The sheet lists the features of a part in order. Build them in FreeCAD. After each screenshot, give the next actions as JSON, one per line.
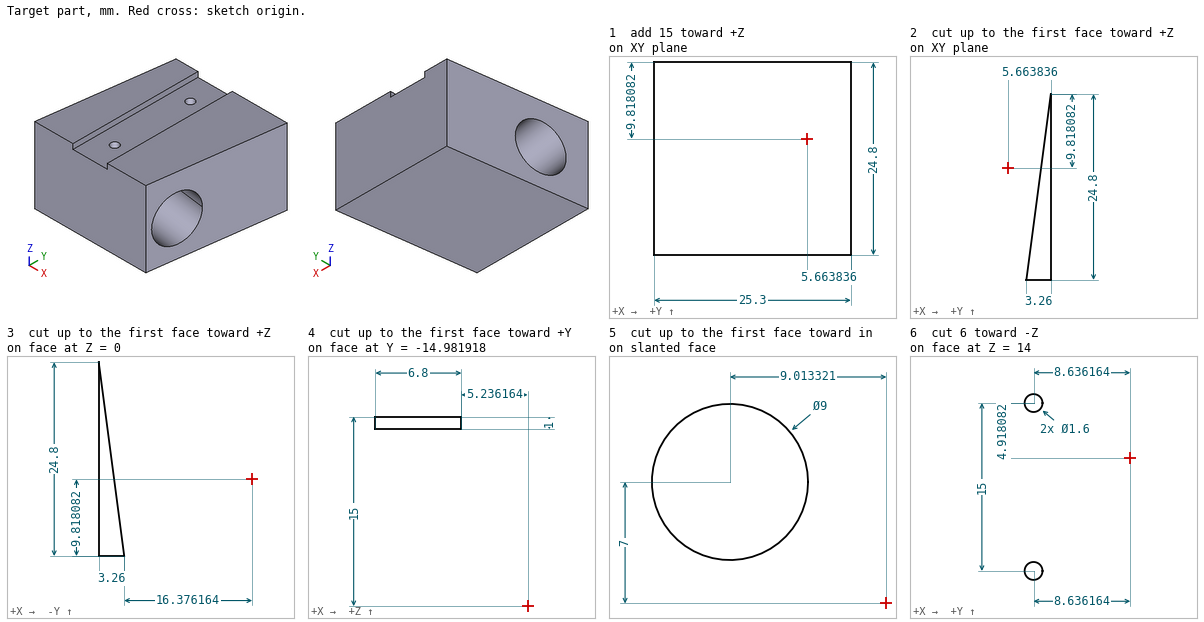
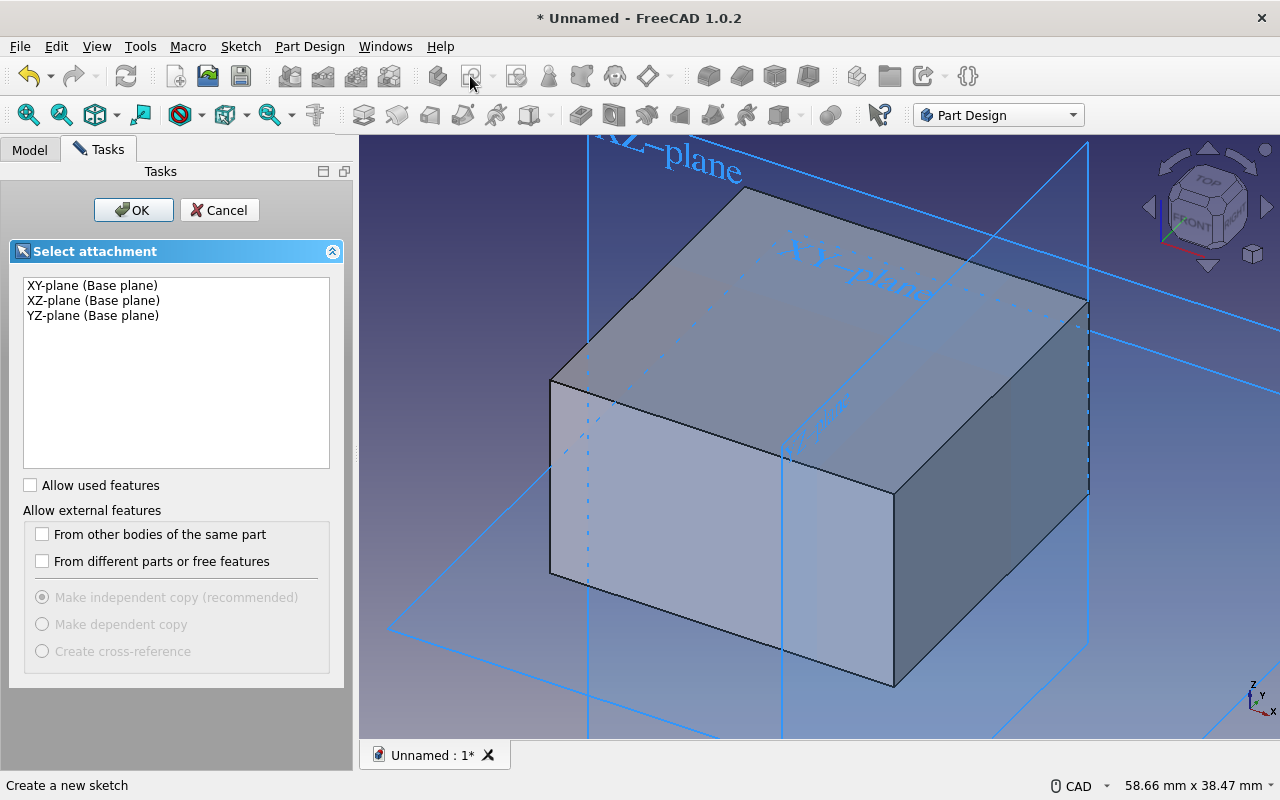
{"action": "left_click", "coordinate": [84, 286]}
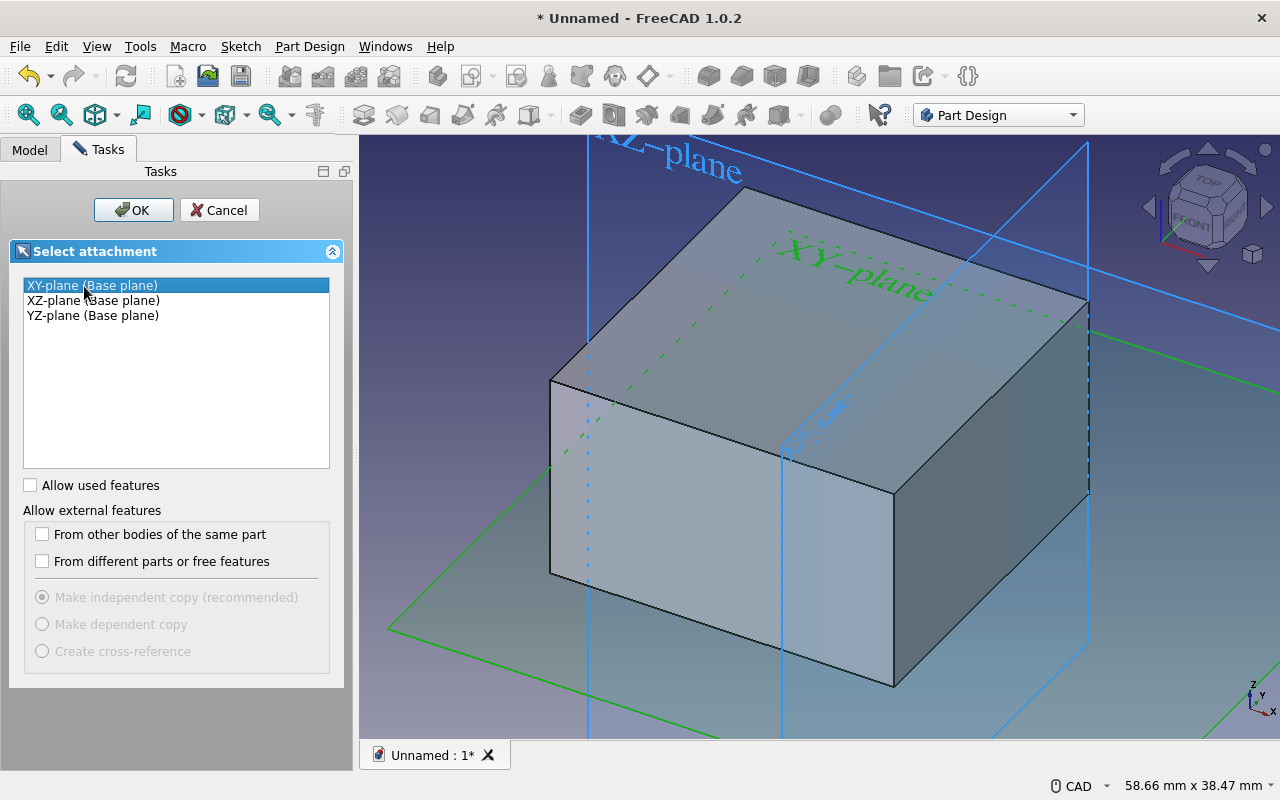
{"action": "left_click", "coordinate": [134, 210]}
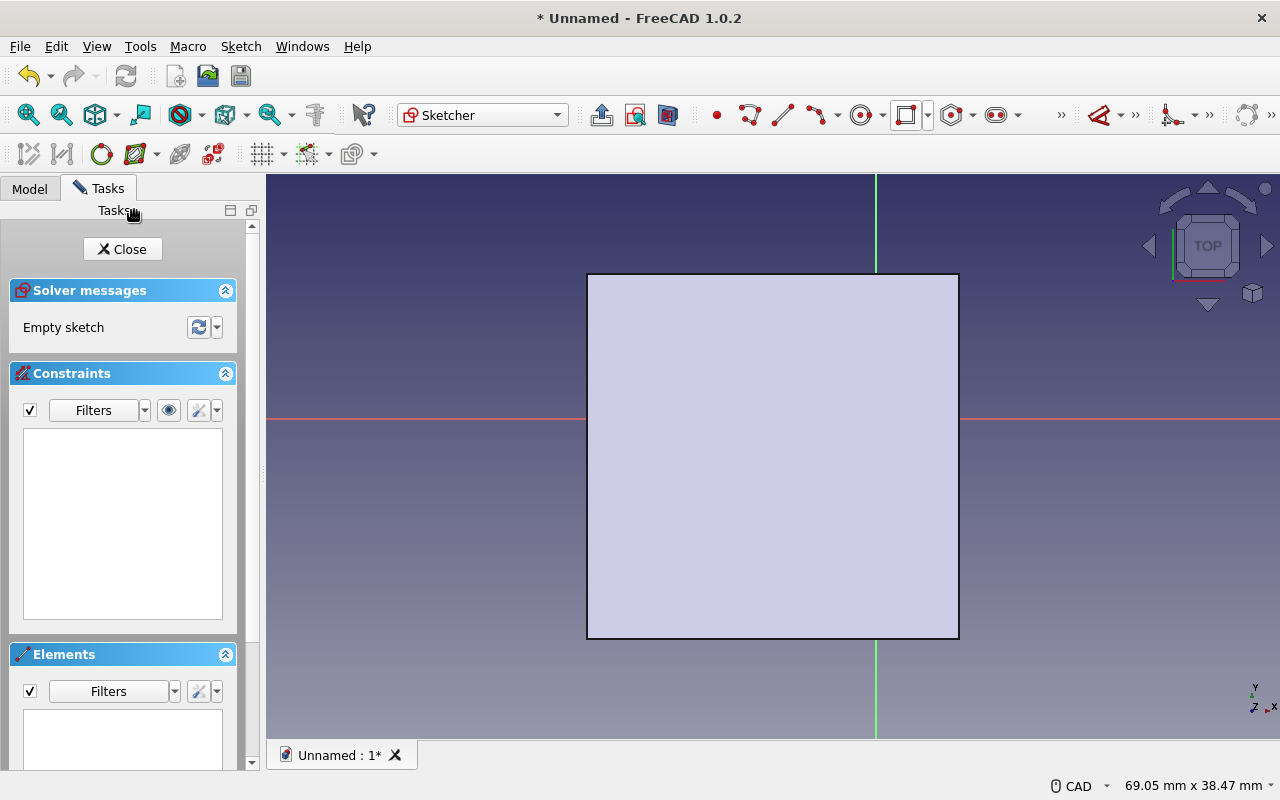
{"action": "left_click", "coordinate": [668, 116]}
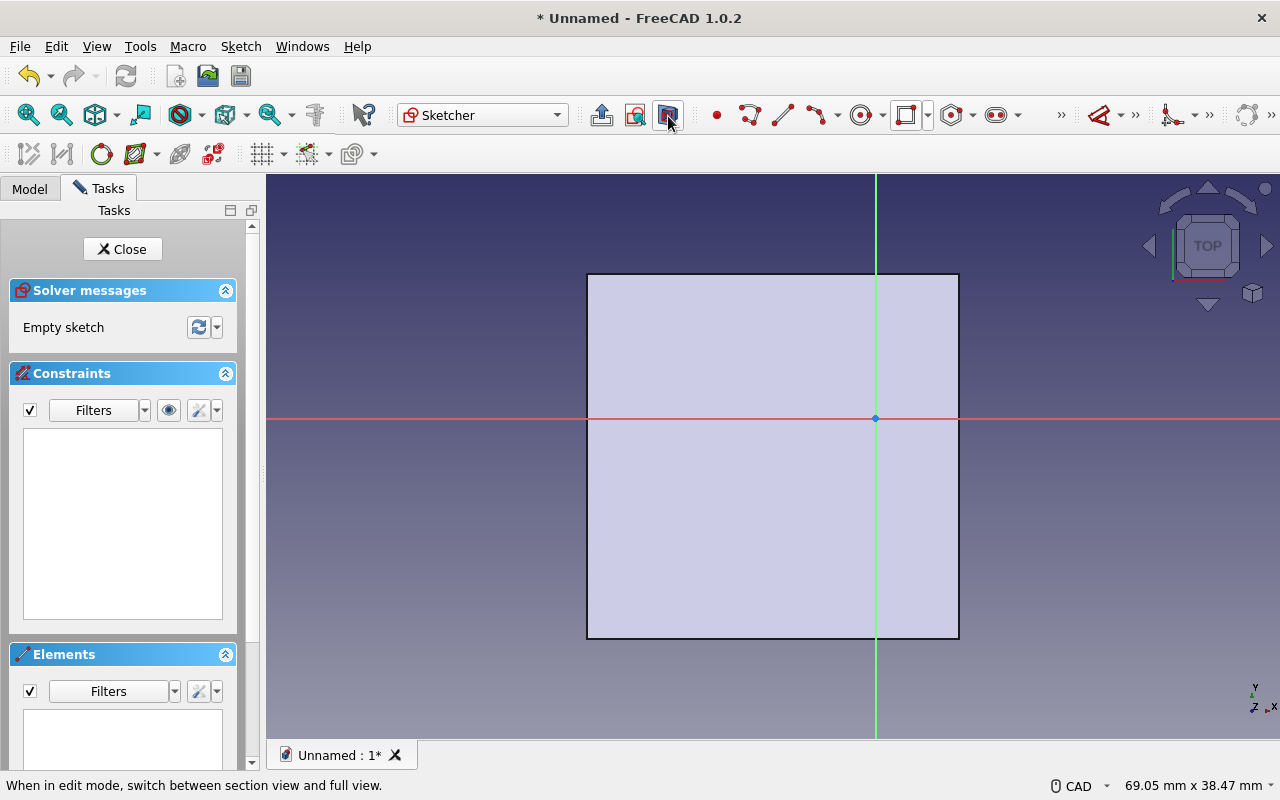
{"action": "left_click", "coordinate": [750, 116]}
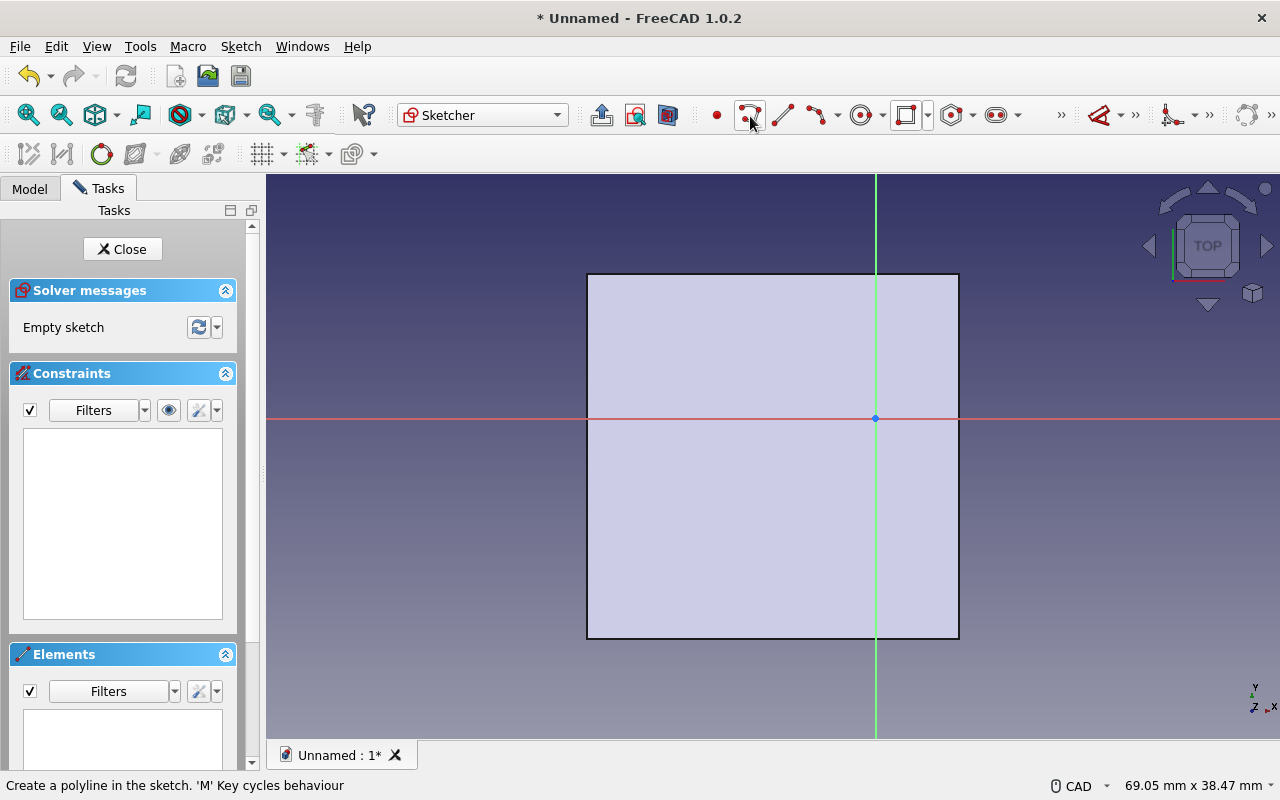
{"action": "left_click", "coordinate": [959, 274]}
{"action": "left_click", "coordinate": [959, 639]}
{"action": "left_click", "coordinate": [911, 639]}
{"action": "left_click", "coordinate": [959, 275]}
{"action": "key", "text": "Escape"}
{"action": "key", "text": "Escape"}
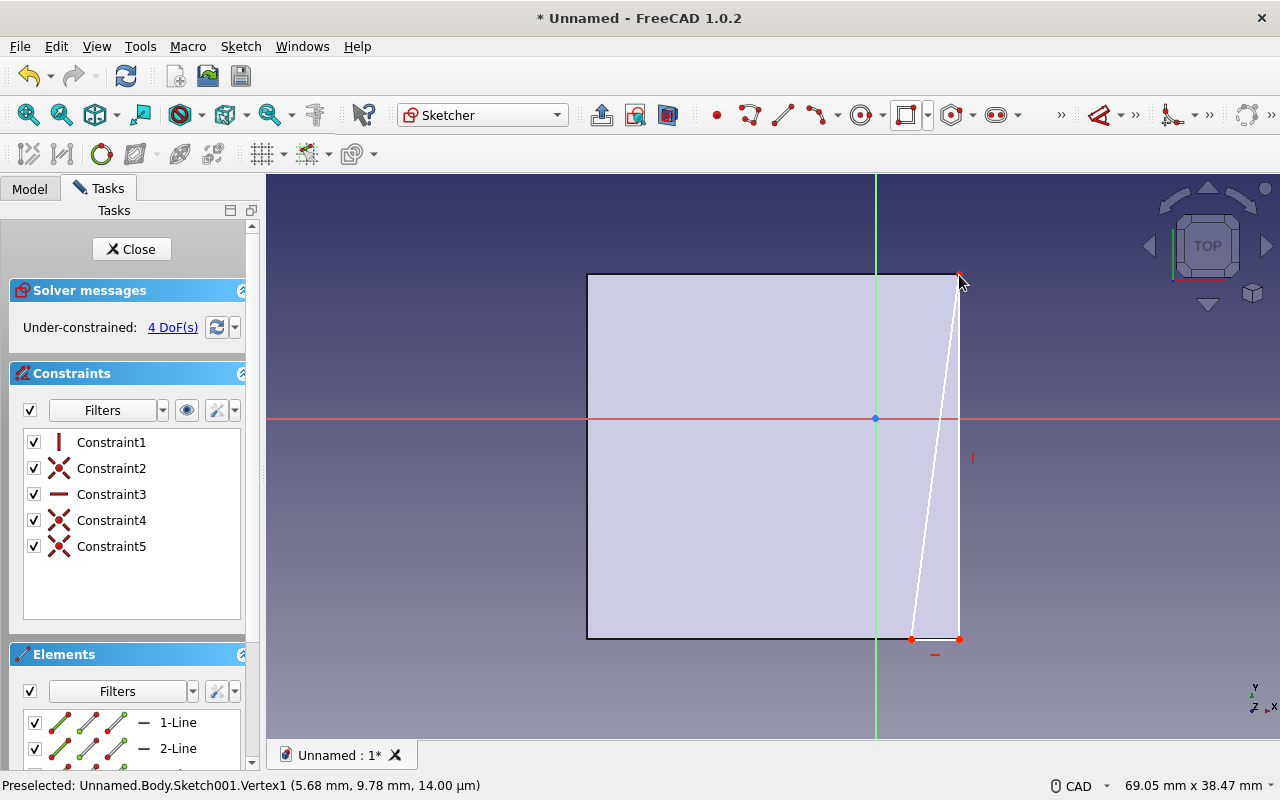
{"action": "left_click", "coordinate": [1098, 116]}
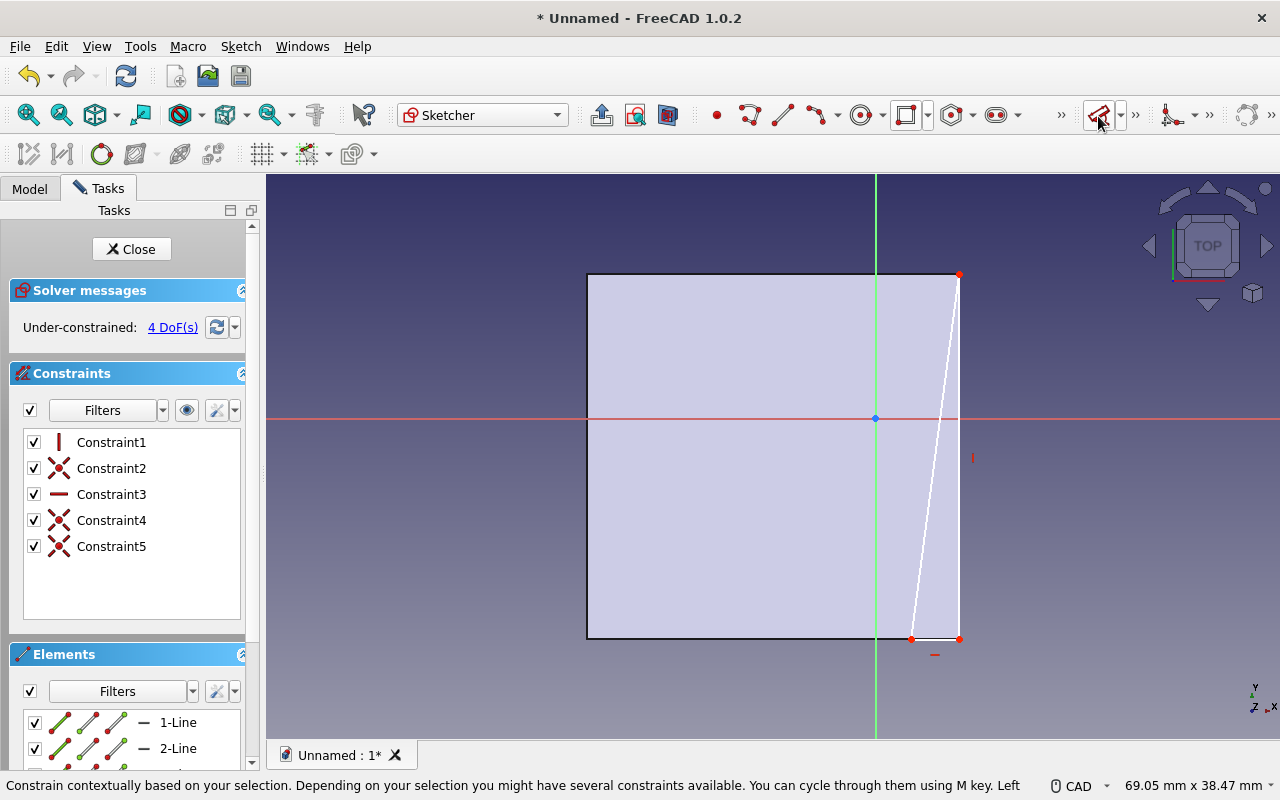
{"action": "left_click", "coordinate": [959, 384]}
{"action": "left_click", "coordinate": [993, 457]}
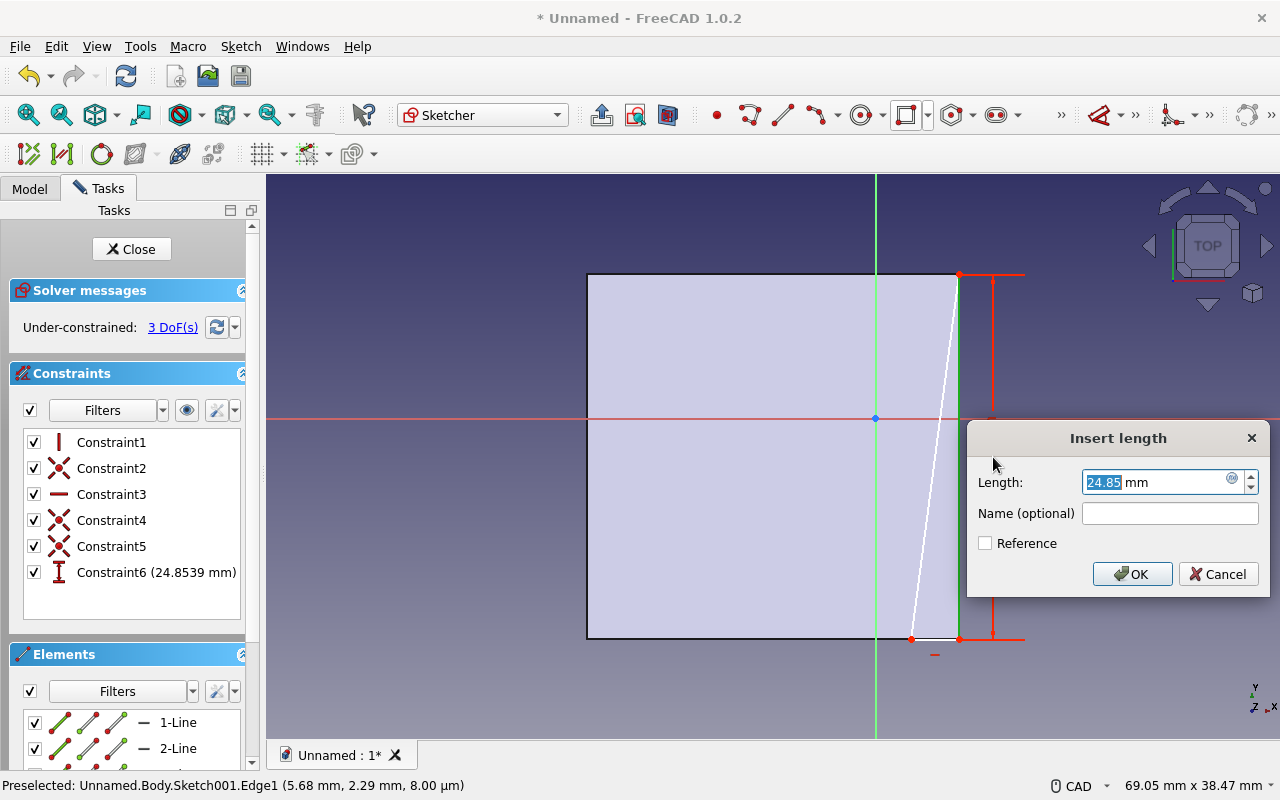
{"action": "type", "text": "24.8"}
{"action": "key", "text": "Return"}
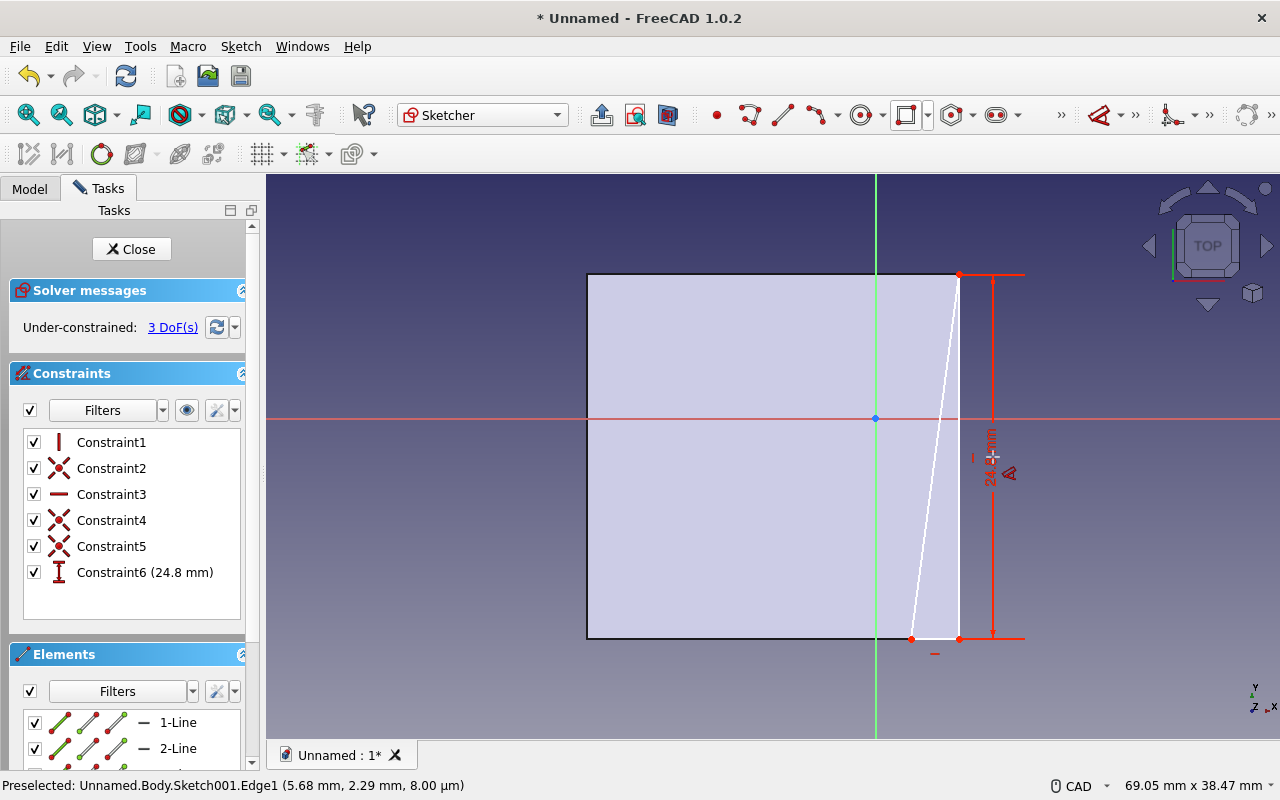
{"action": "left_click", "coordinate": [945, 639]}
{"action": "left_click", "coordinate": [935, 673]}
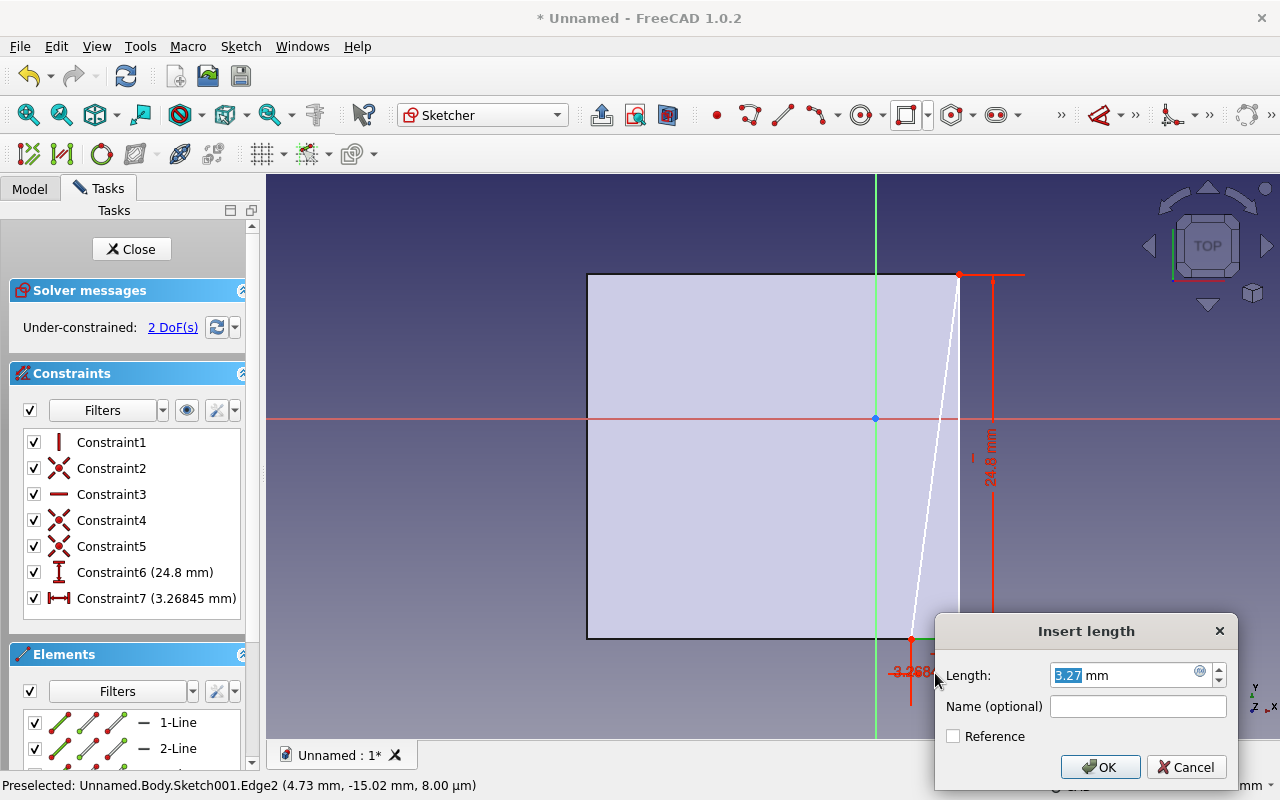
{"action": "type", "text": "3.26"}
{"action": "key", "text": "Return"}